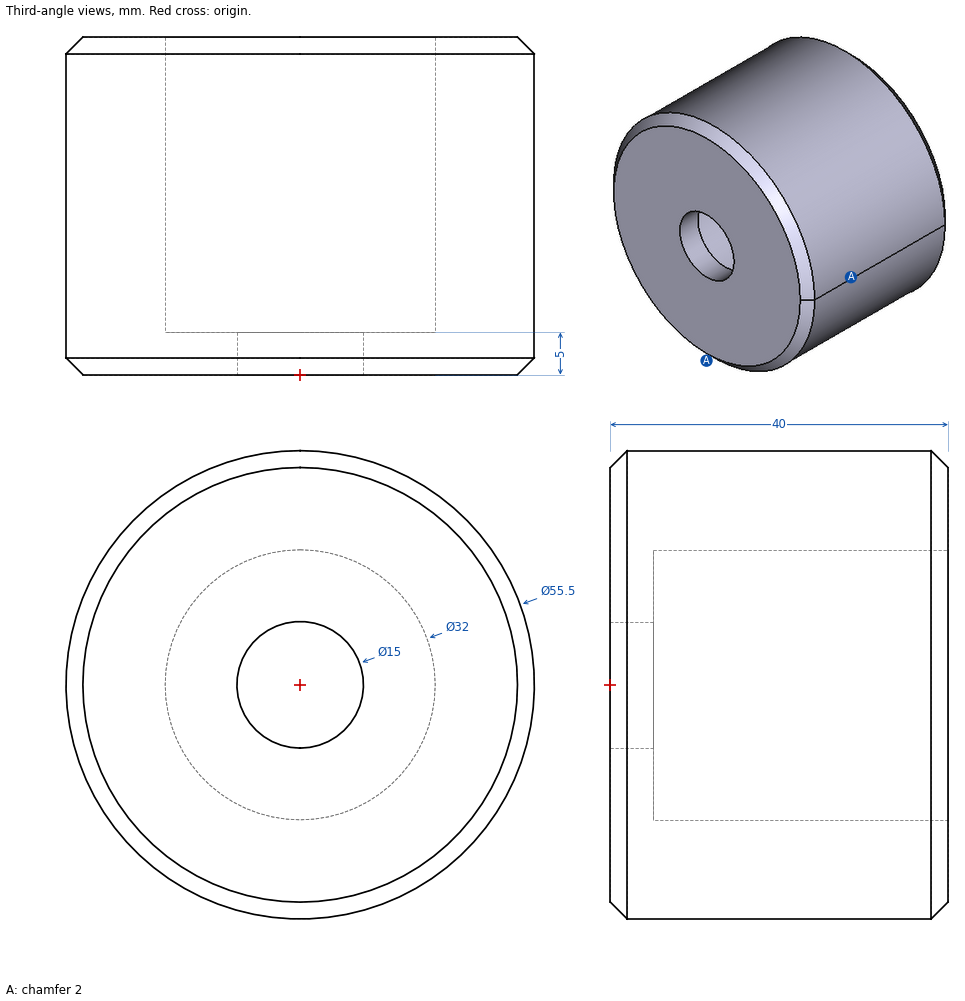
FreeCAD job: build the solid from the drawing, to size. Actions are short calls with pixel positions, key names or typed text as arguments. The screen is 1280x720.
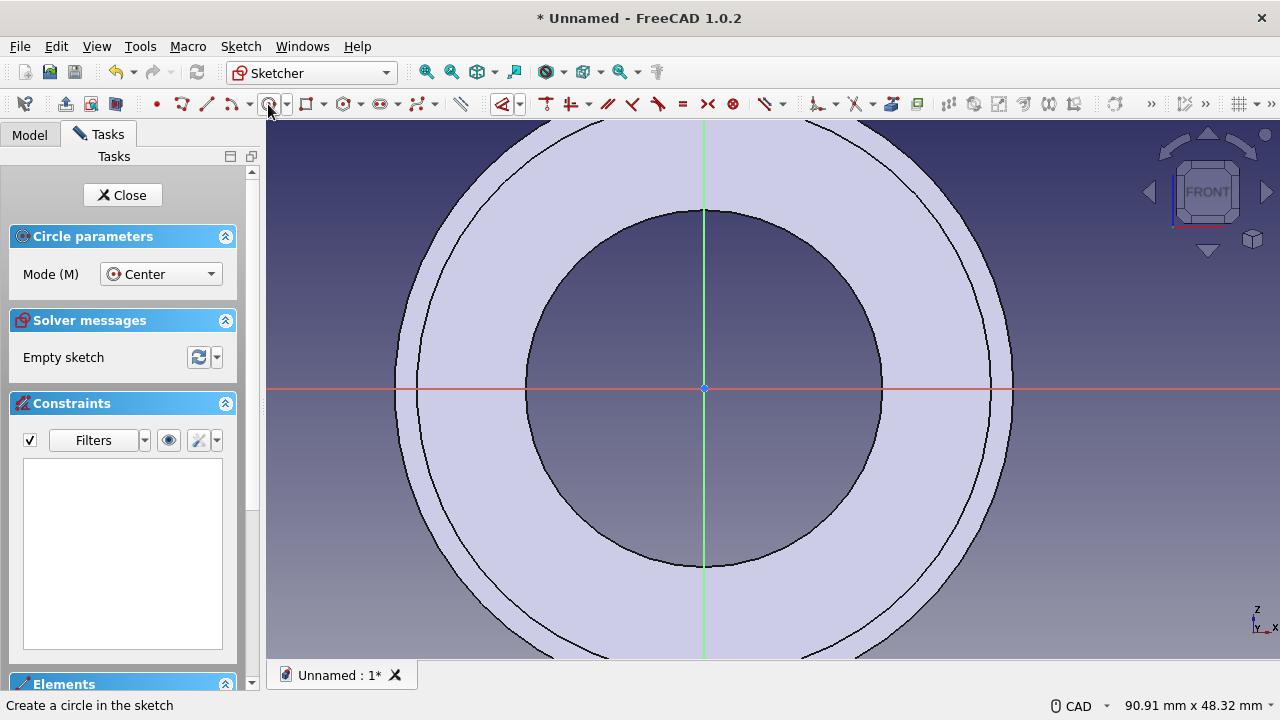
click(704, 389)
click(830, 262)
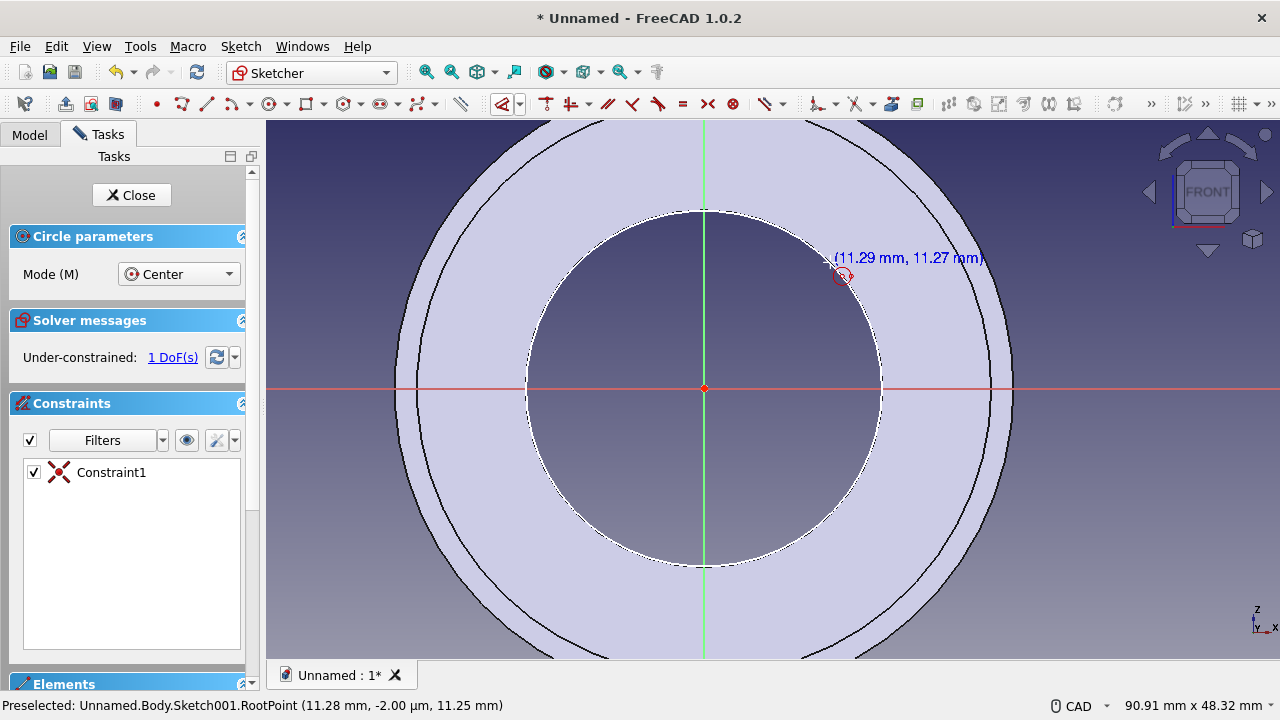
click(704, 389)
click(763, 330)
key(Escape)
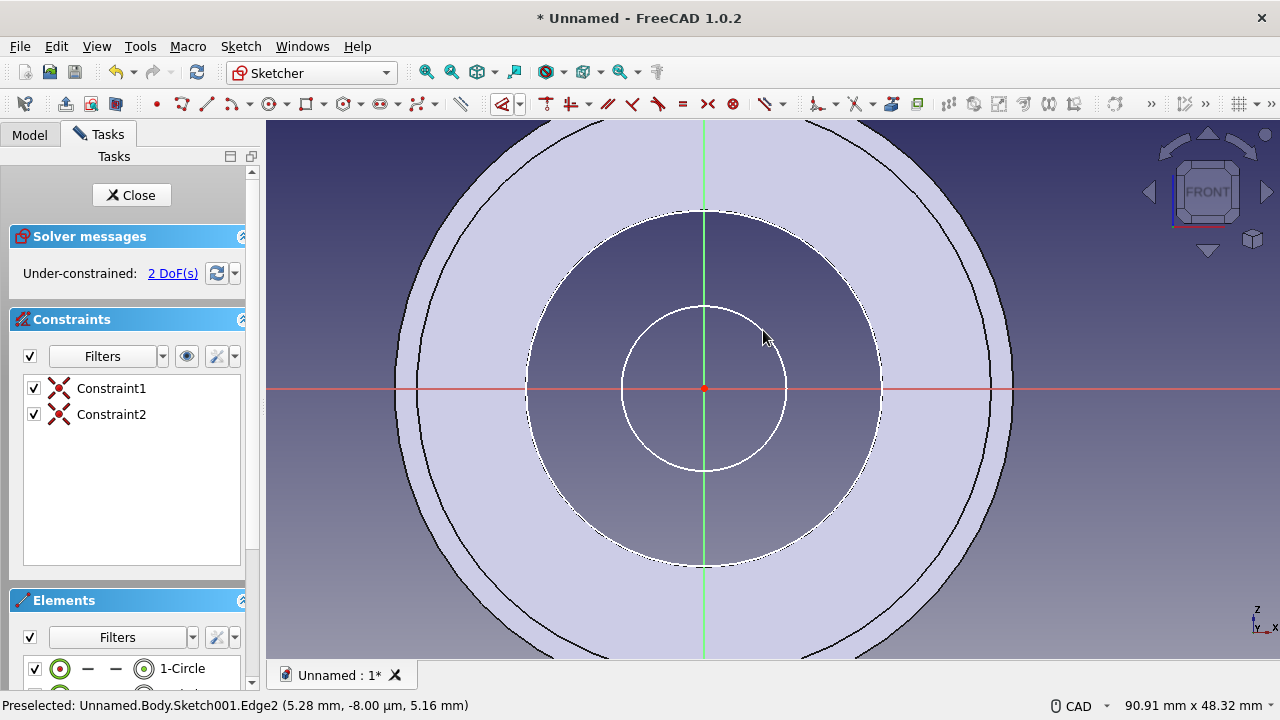
click(829, 262)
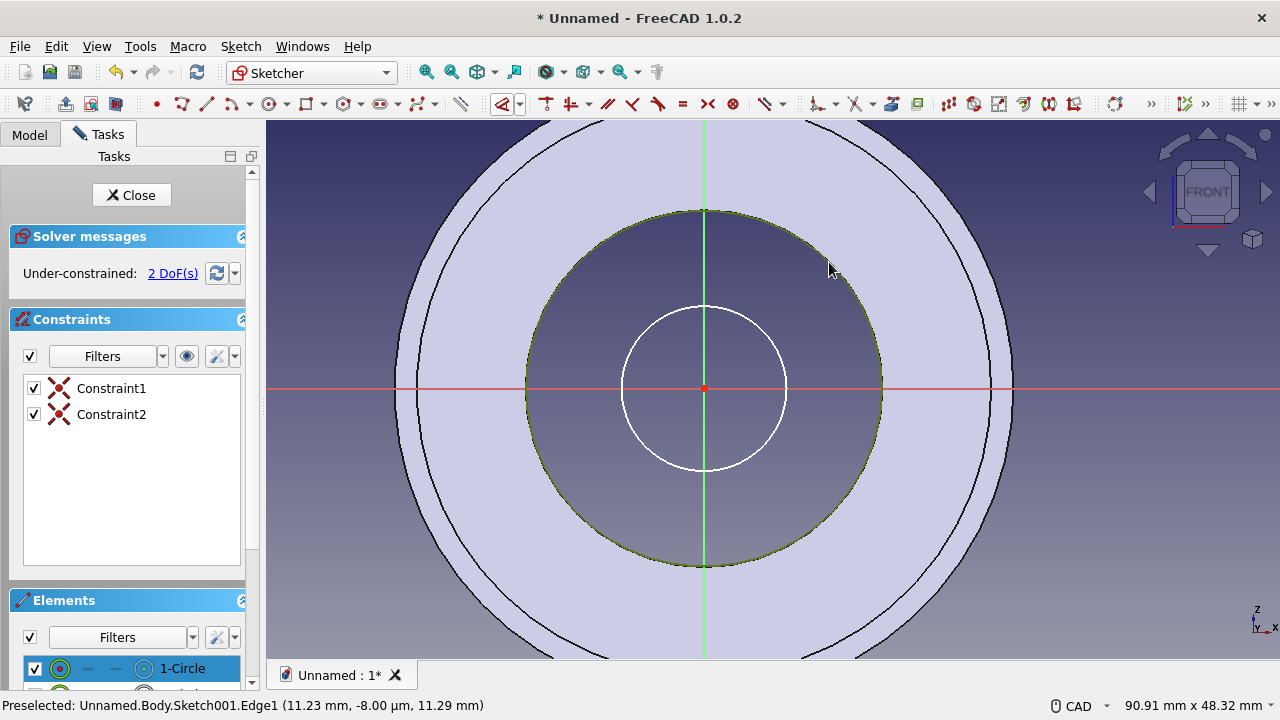
key(k)
key(o)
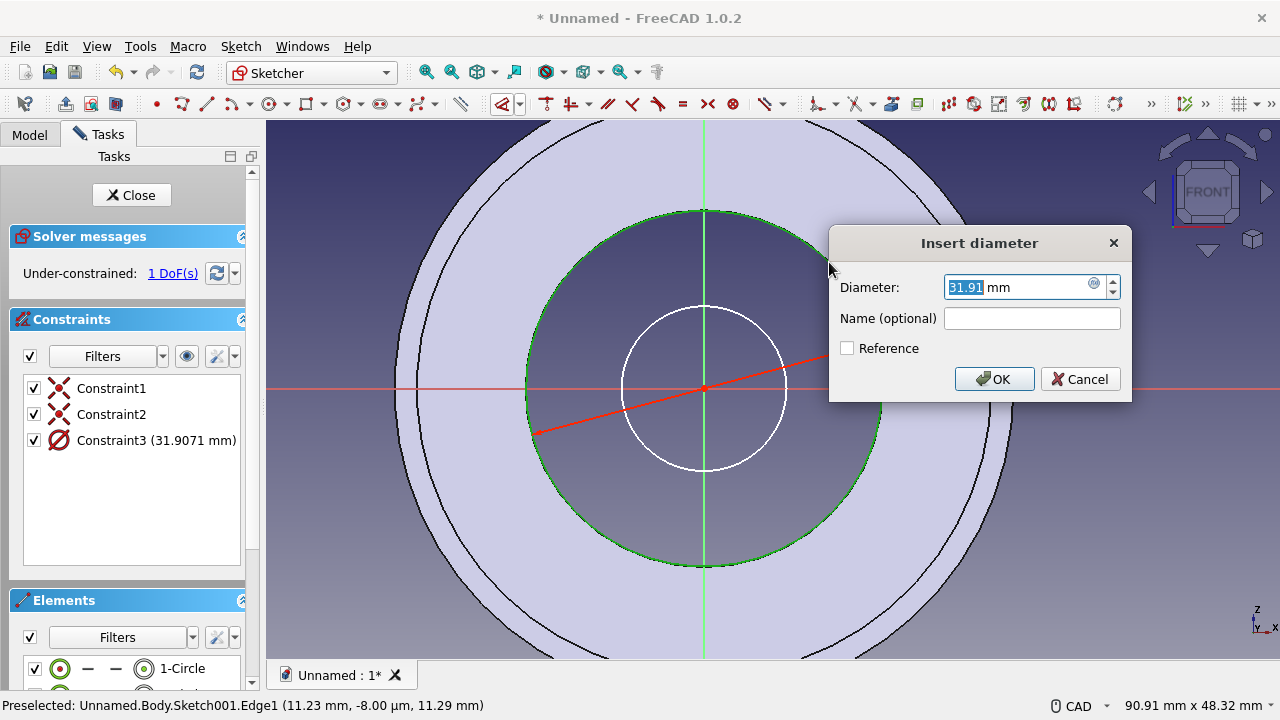
text(32)
key(Return)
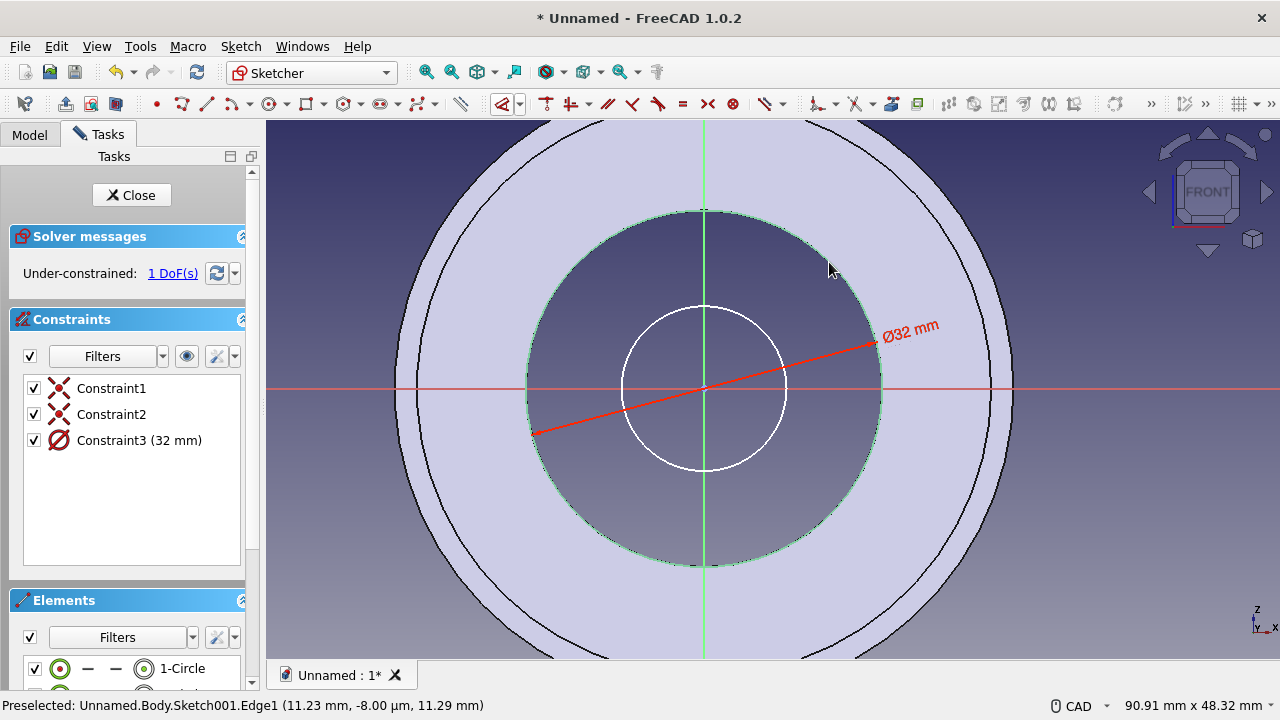
click(762, 330)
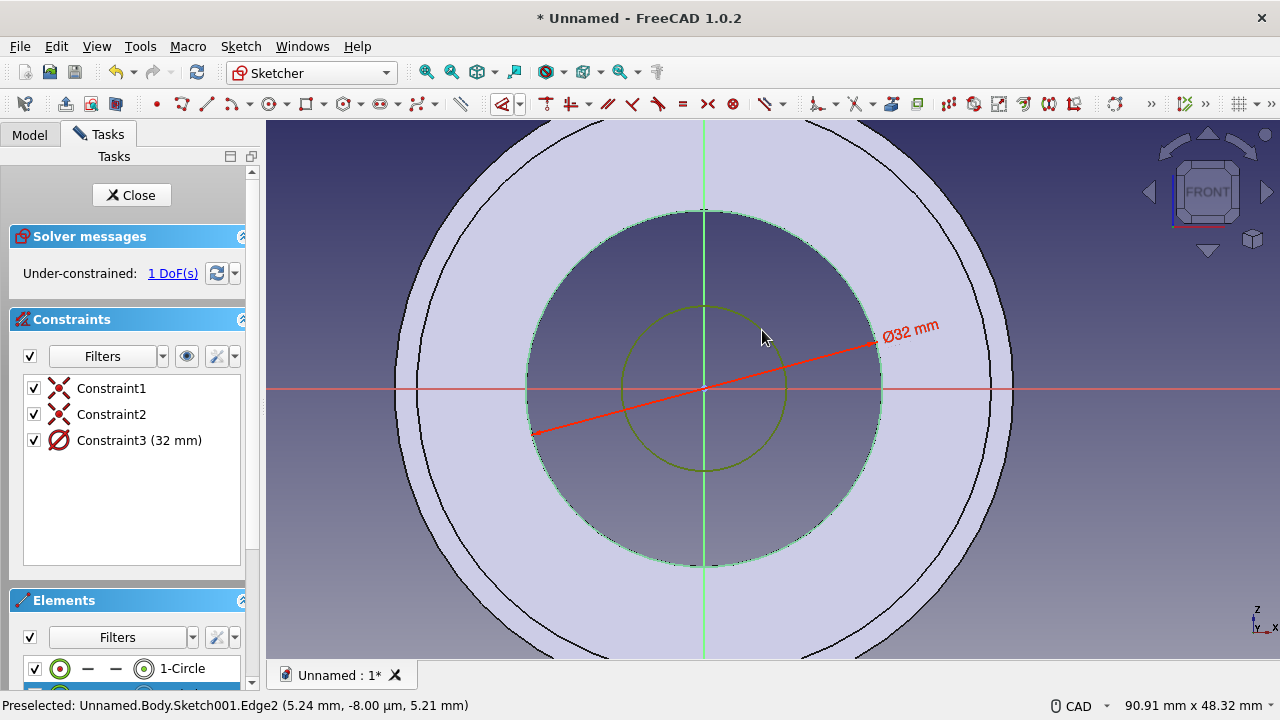
click(520, 104)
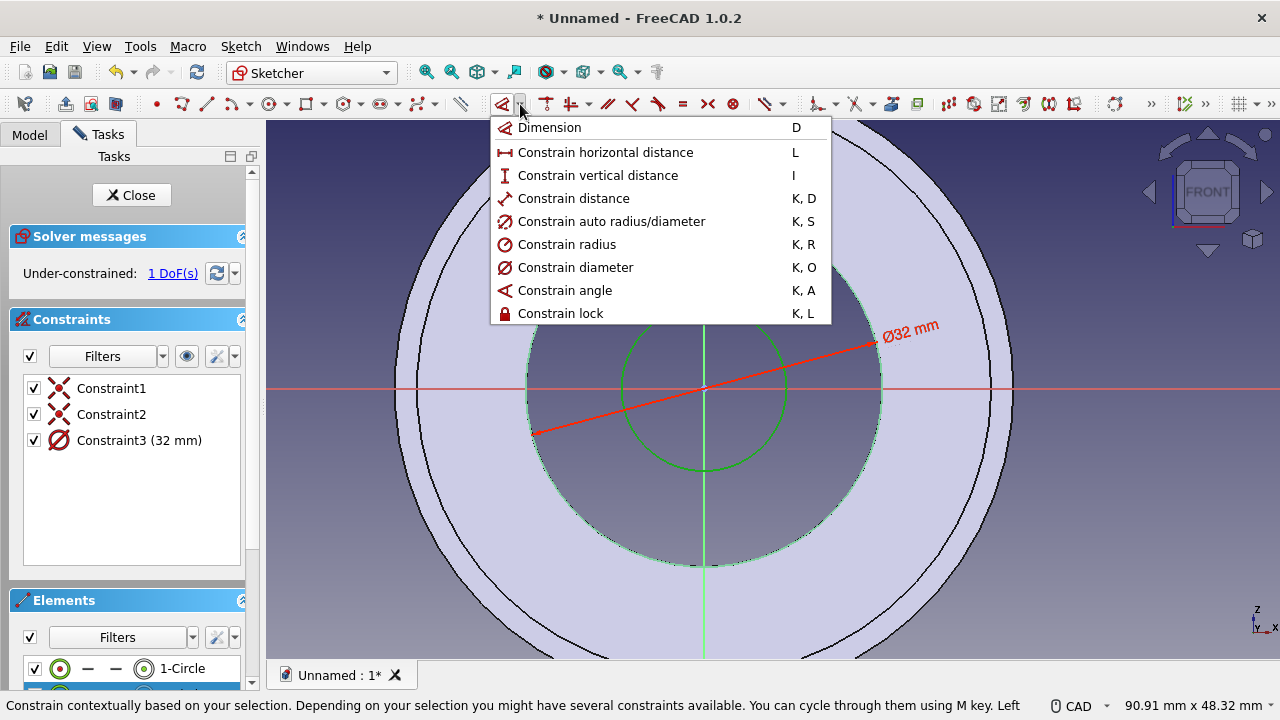
click(661, 268)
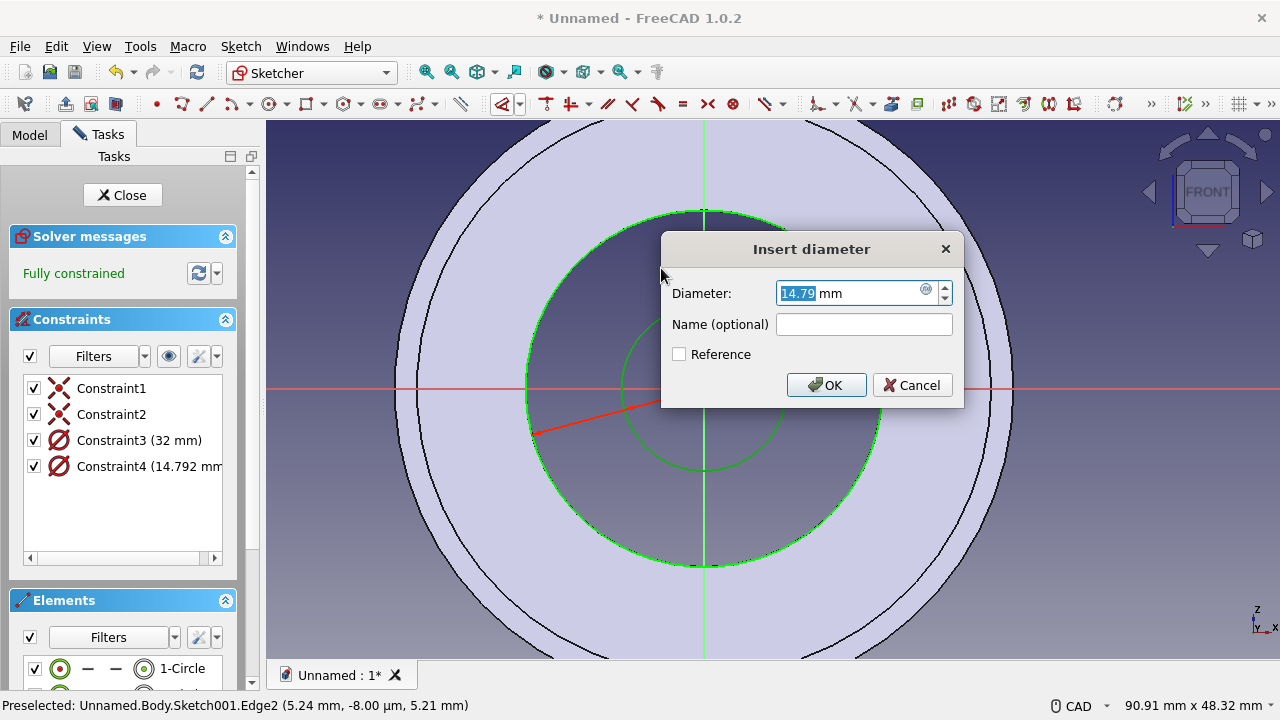
text(15)
key(Return)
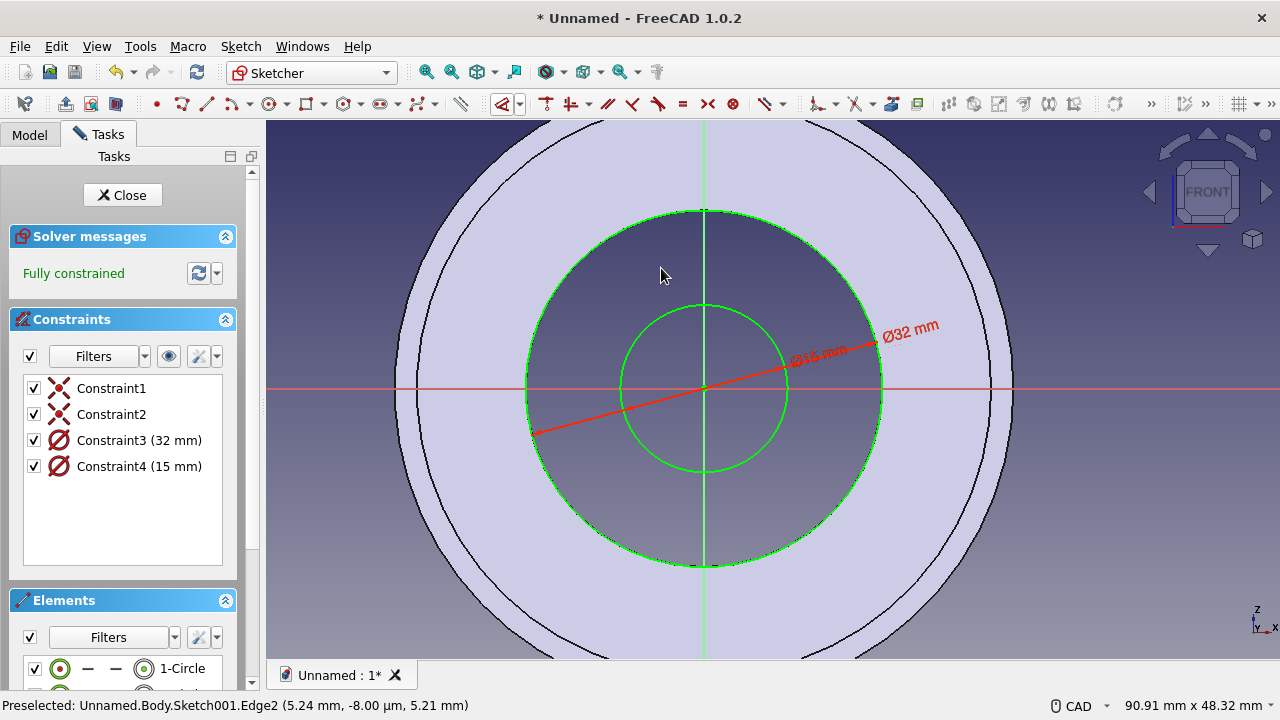
click(123, 195)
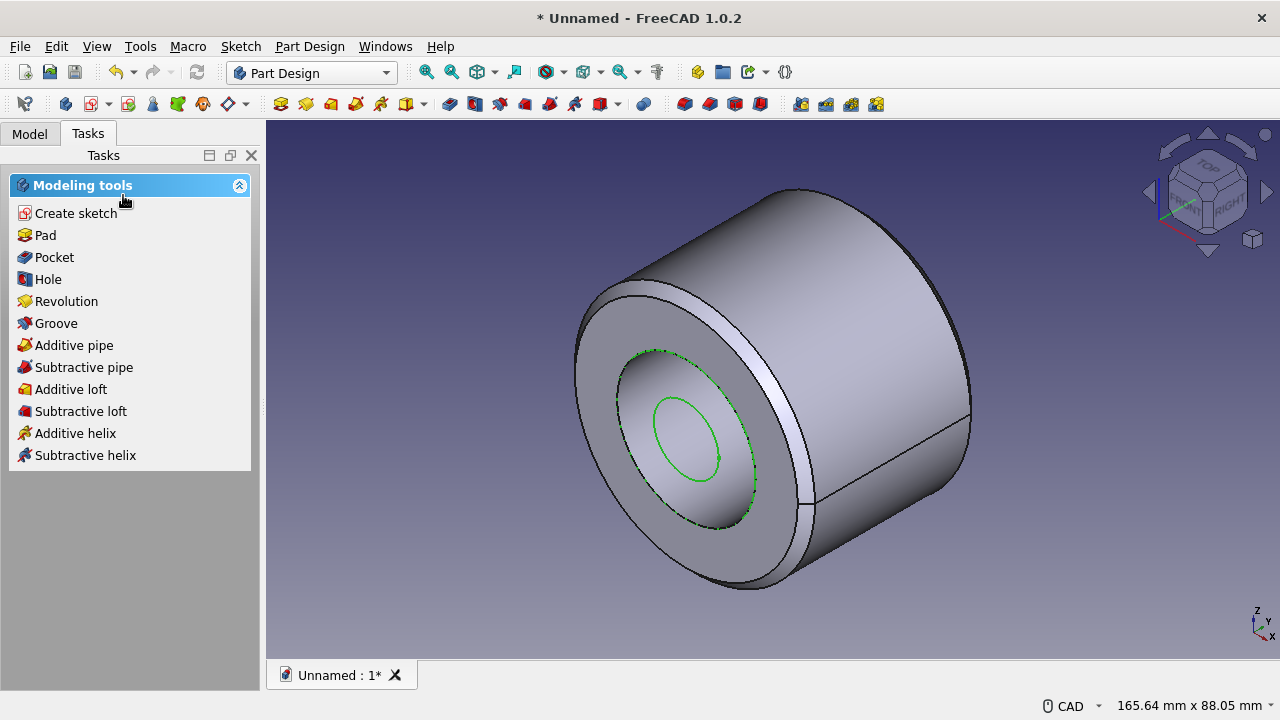
click(281, 104)